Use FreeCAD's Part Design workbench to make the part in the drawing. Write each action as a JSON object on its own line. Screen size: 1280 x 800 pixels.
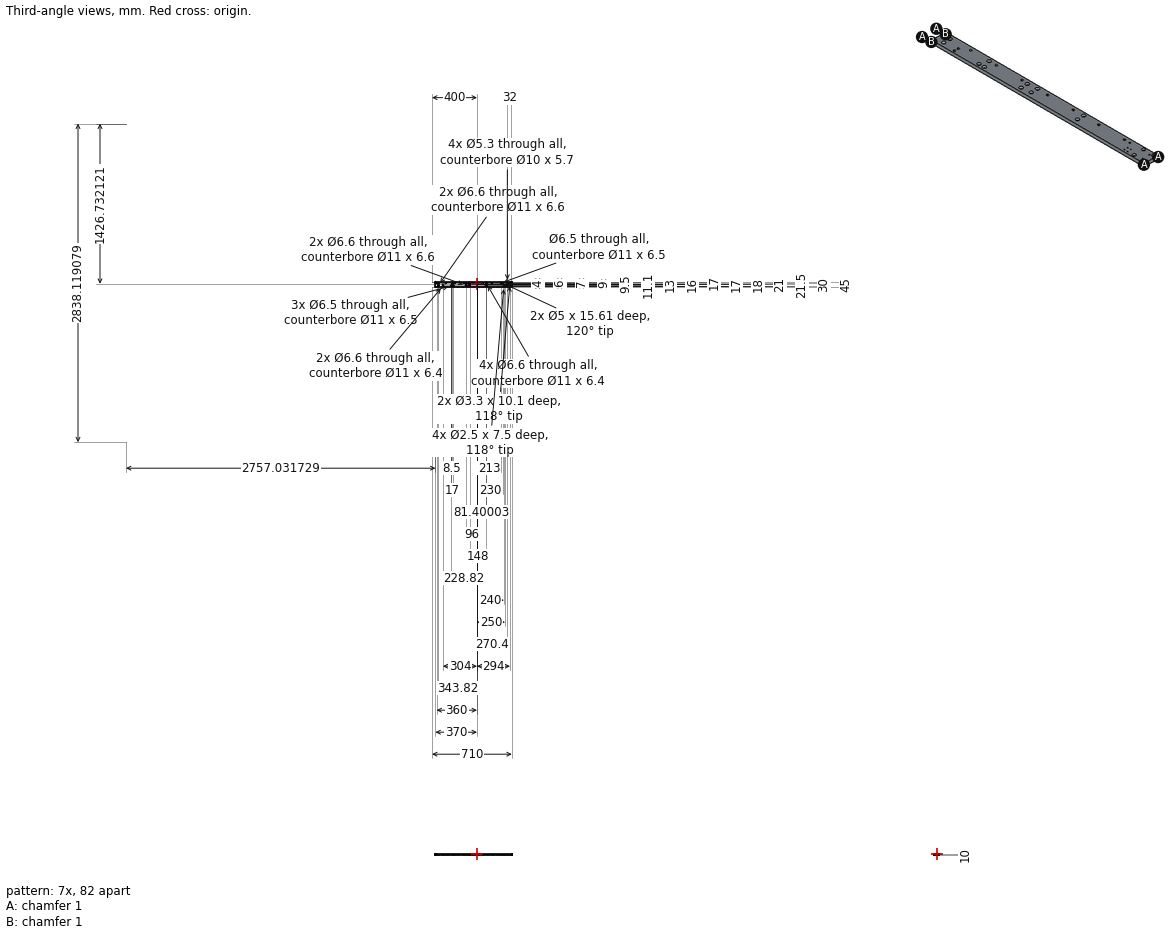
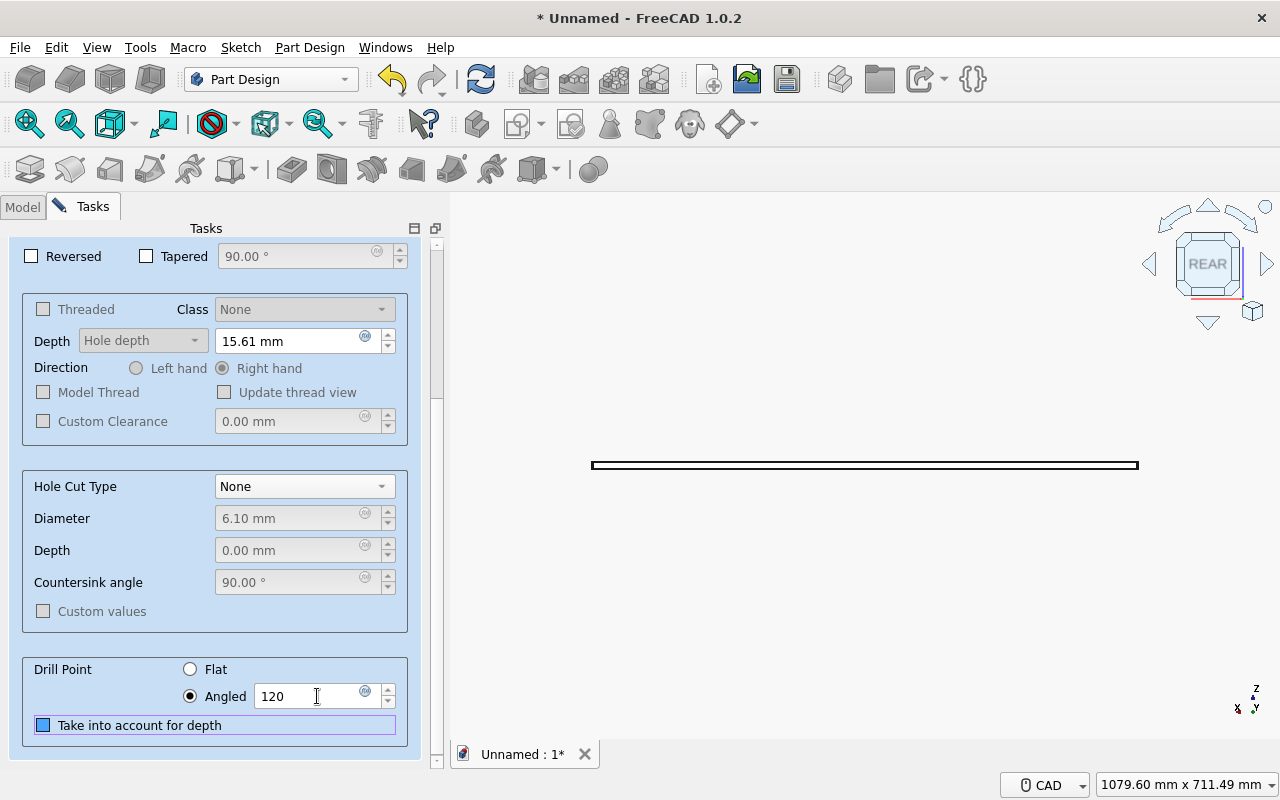
{"action": "scroll", "coordinate": [437, 503], "scroll_direction": "up", "scroll_amount": 5}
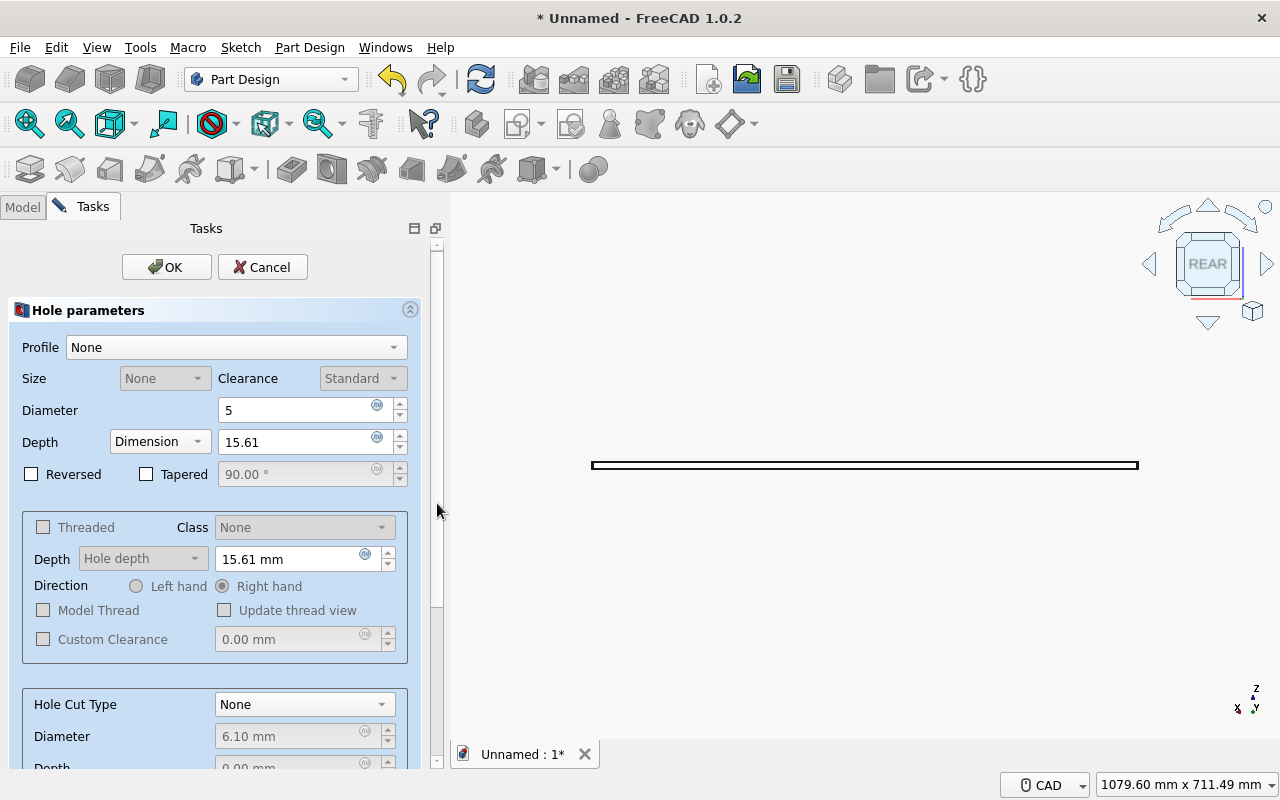
{"action": "left_click", "coordinate": [167, 267]}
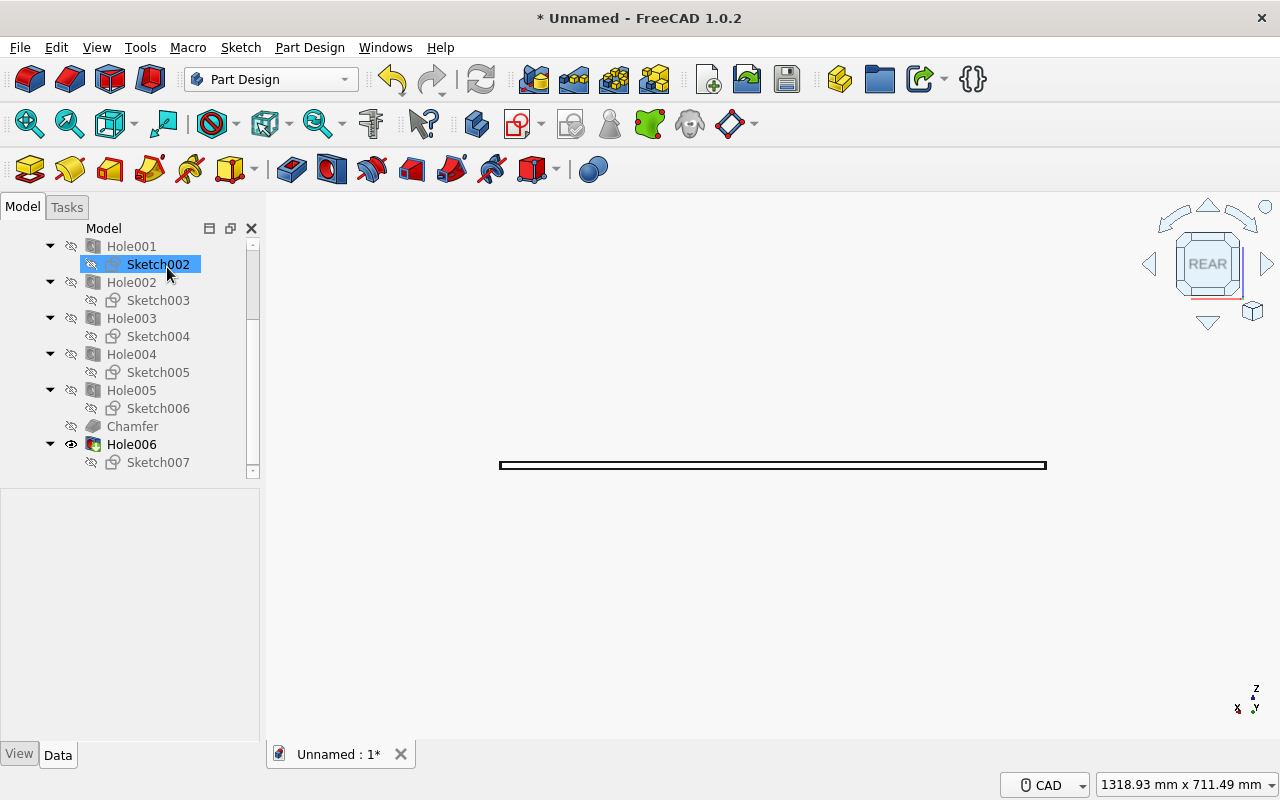
{"action": "left_click", "coordinate": [518, 124]}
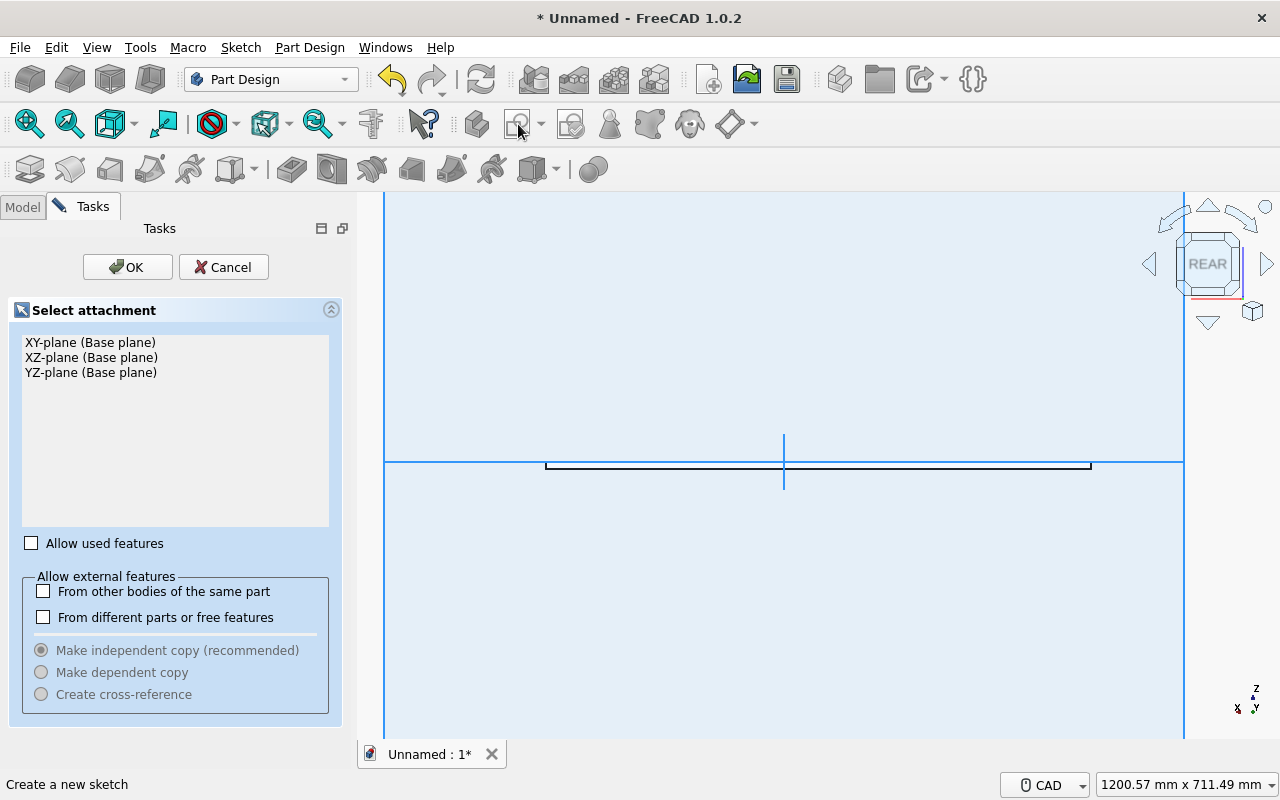
{"action": "left_click", "coordinate": [82, 342]}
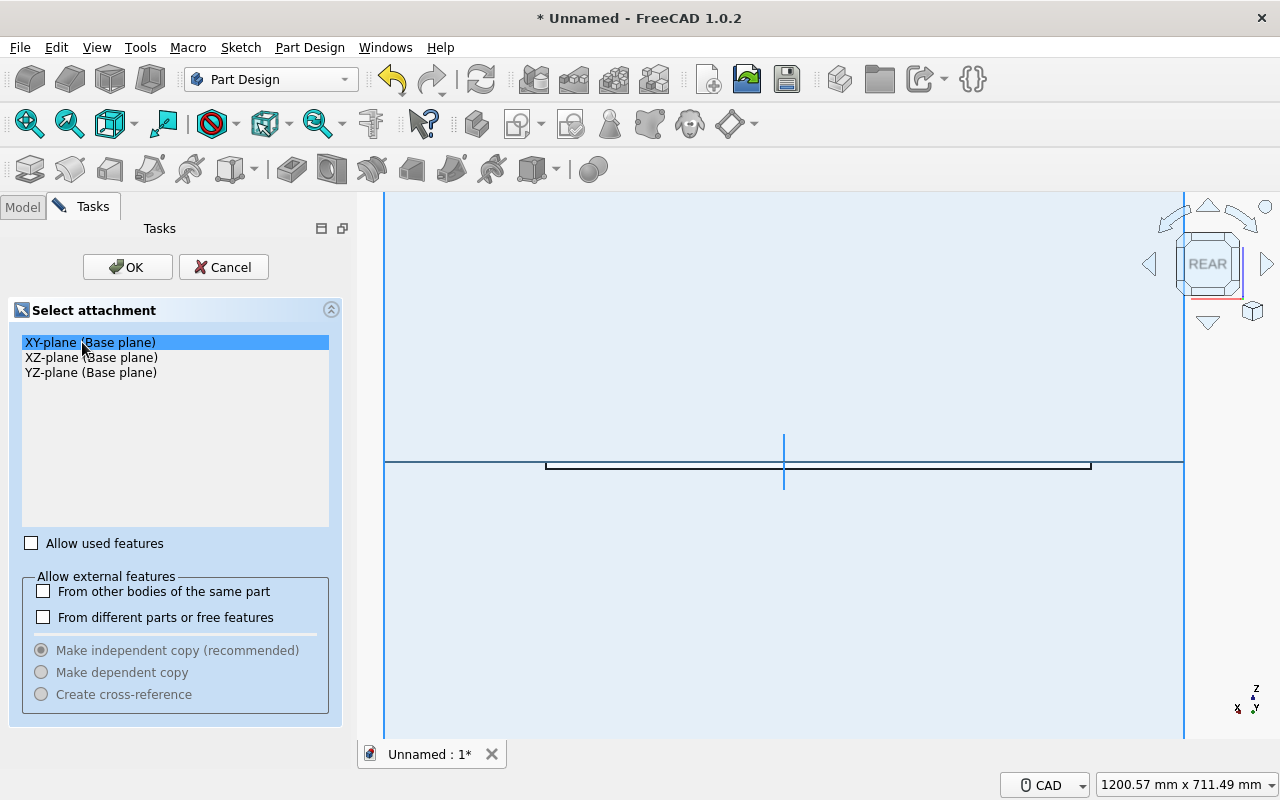
{"action": "left_click", "coordinate": [128, 267]}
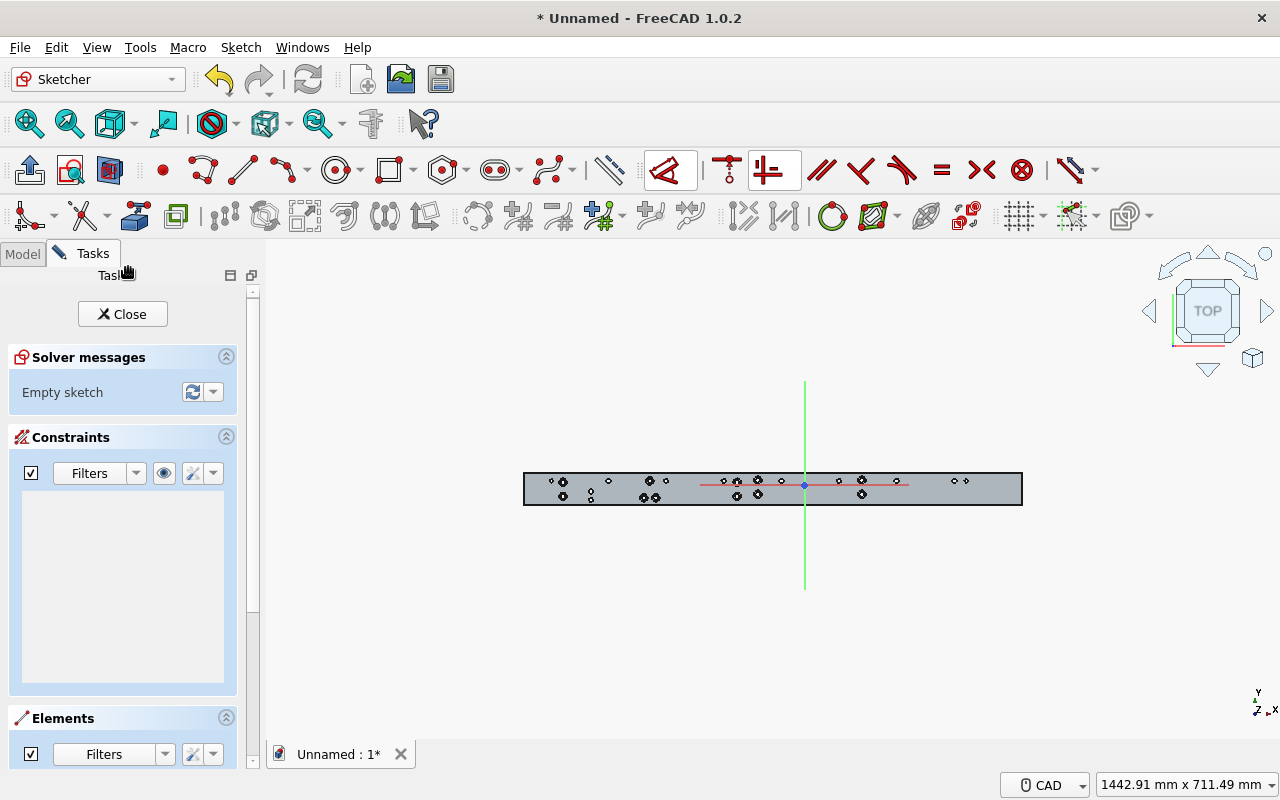
{"action": "scroll", "coordinate": [1030, 489], "scroll_direction": "up", "scroll_amount": 13}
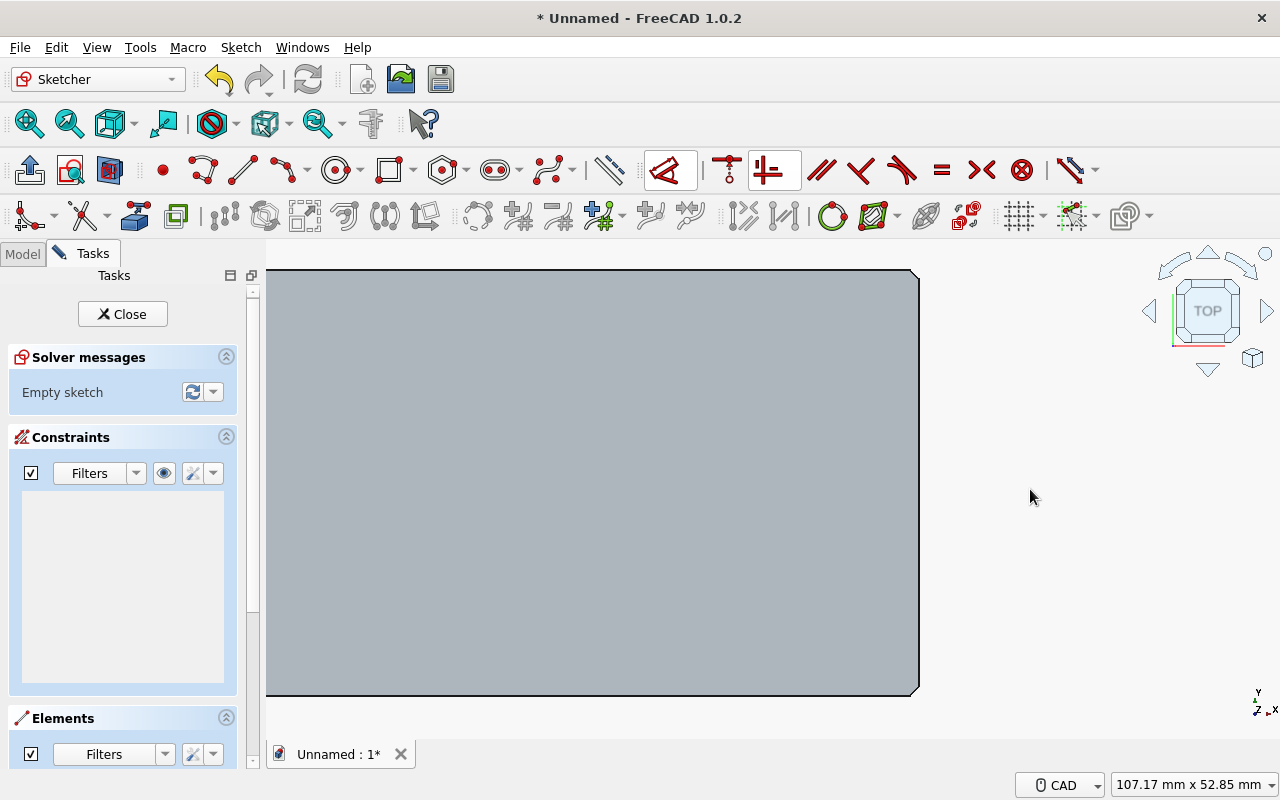
{"action": "left_click", "coordinate": [336, 170]}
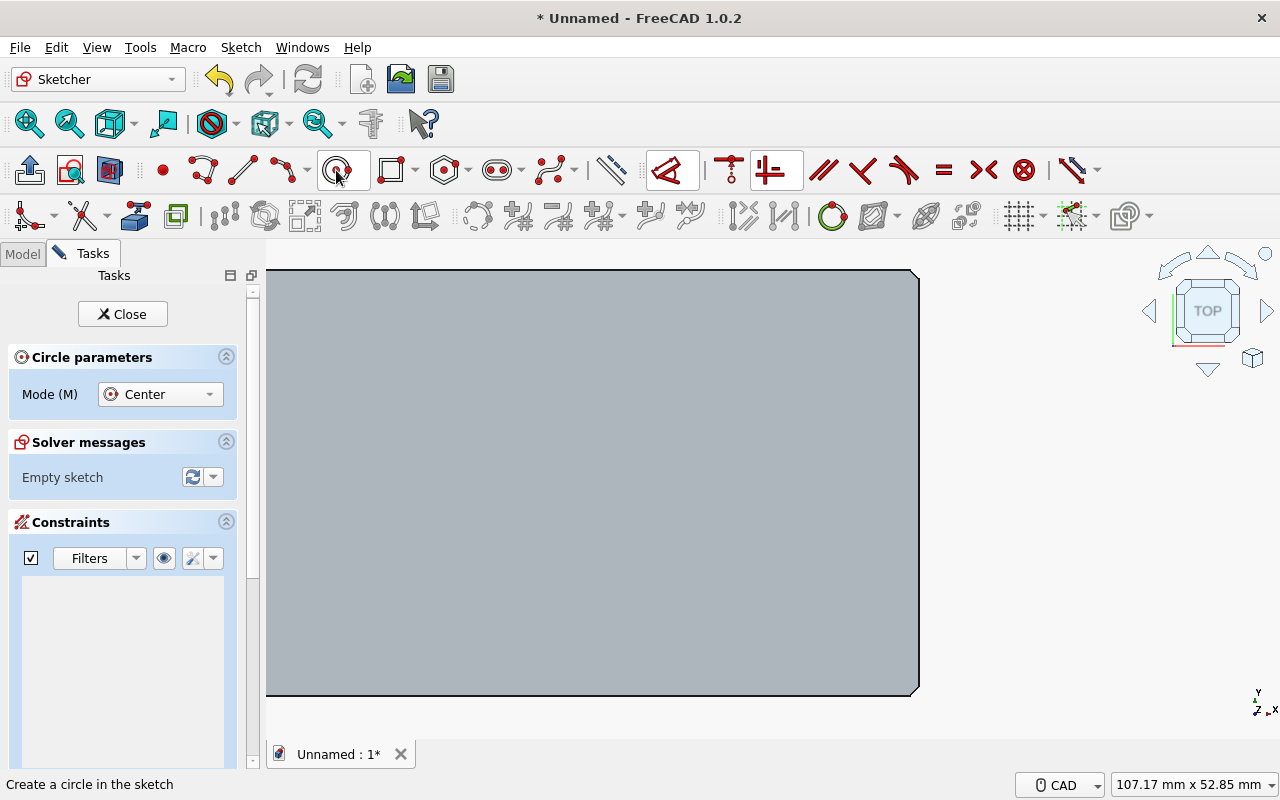
{"action": "left_click", "coordinate": [545, 341]}
{"action": "left_click", "coordinate": [562, 323]}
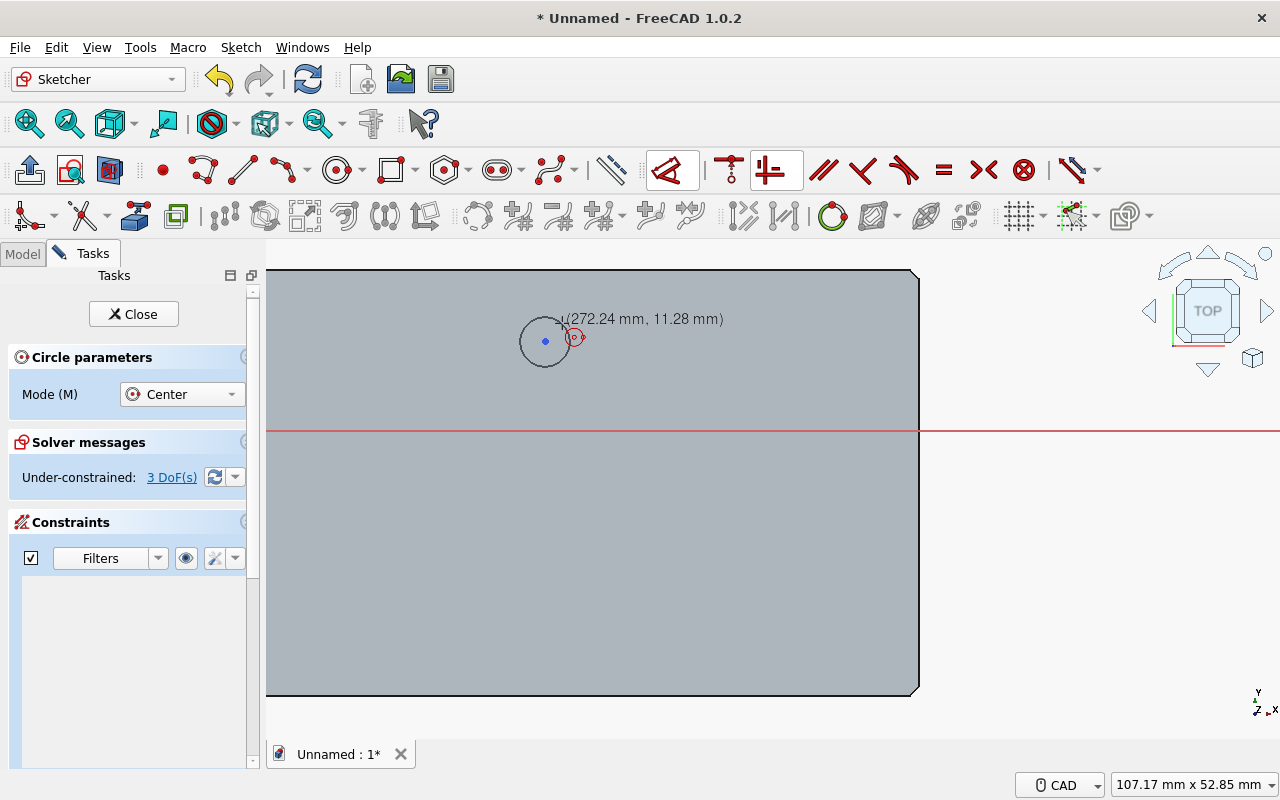
{"action": "left_click", "coordinate": [847, 341]}
{"action": "left_click", "coordinate": [865, 323]}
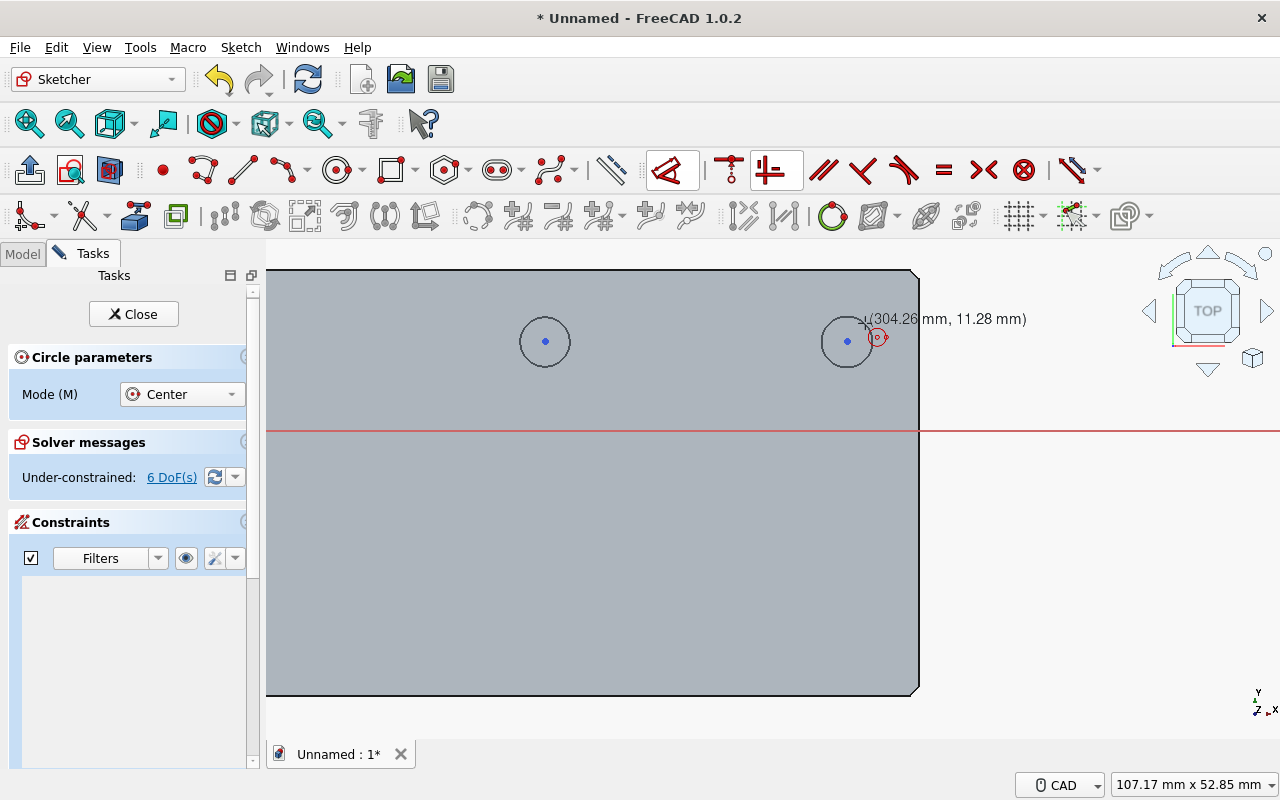
{"action": "left_click", "coordinate": [545, 625]}
{"action": "left_click", "coordinate": [562, 607]}